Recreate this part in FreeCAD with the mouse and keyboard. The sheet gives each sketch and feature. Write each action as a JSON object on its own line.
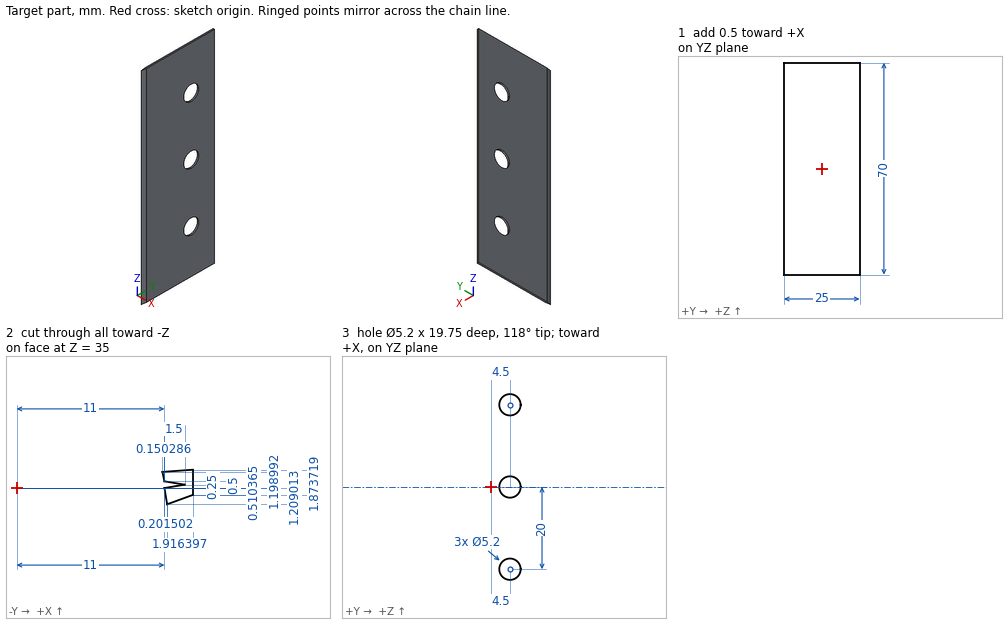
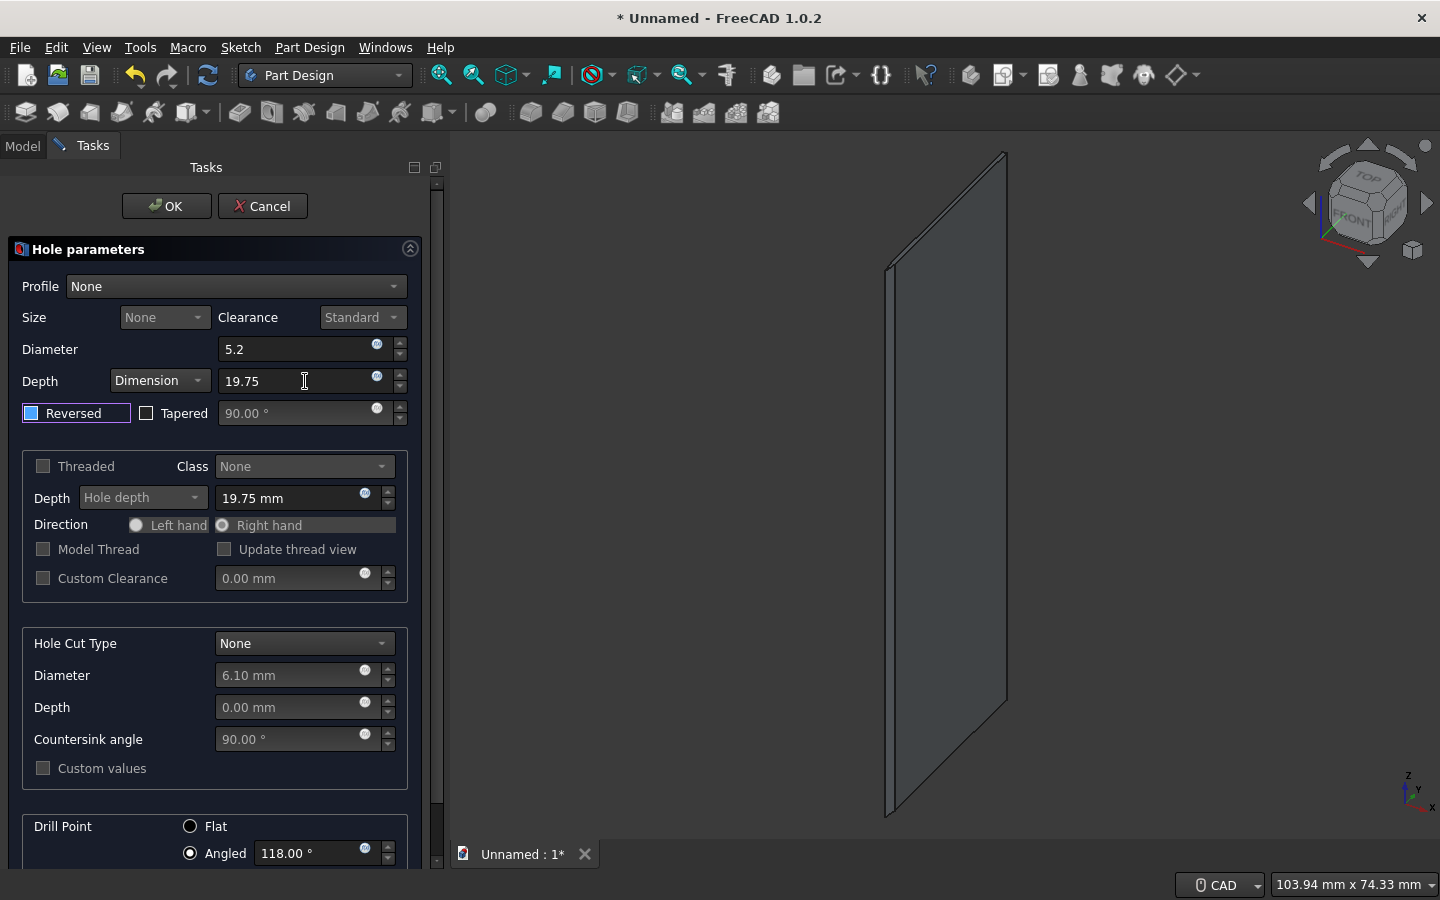
{"action": "left_click", "coordinate": [30, 413]}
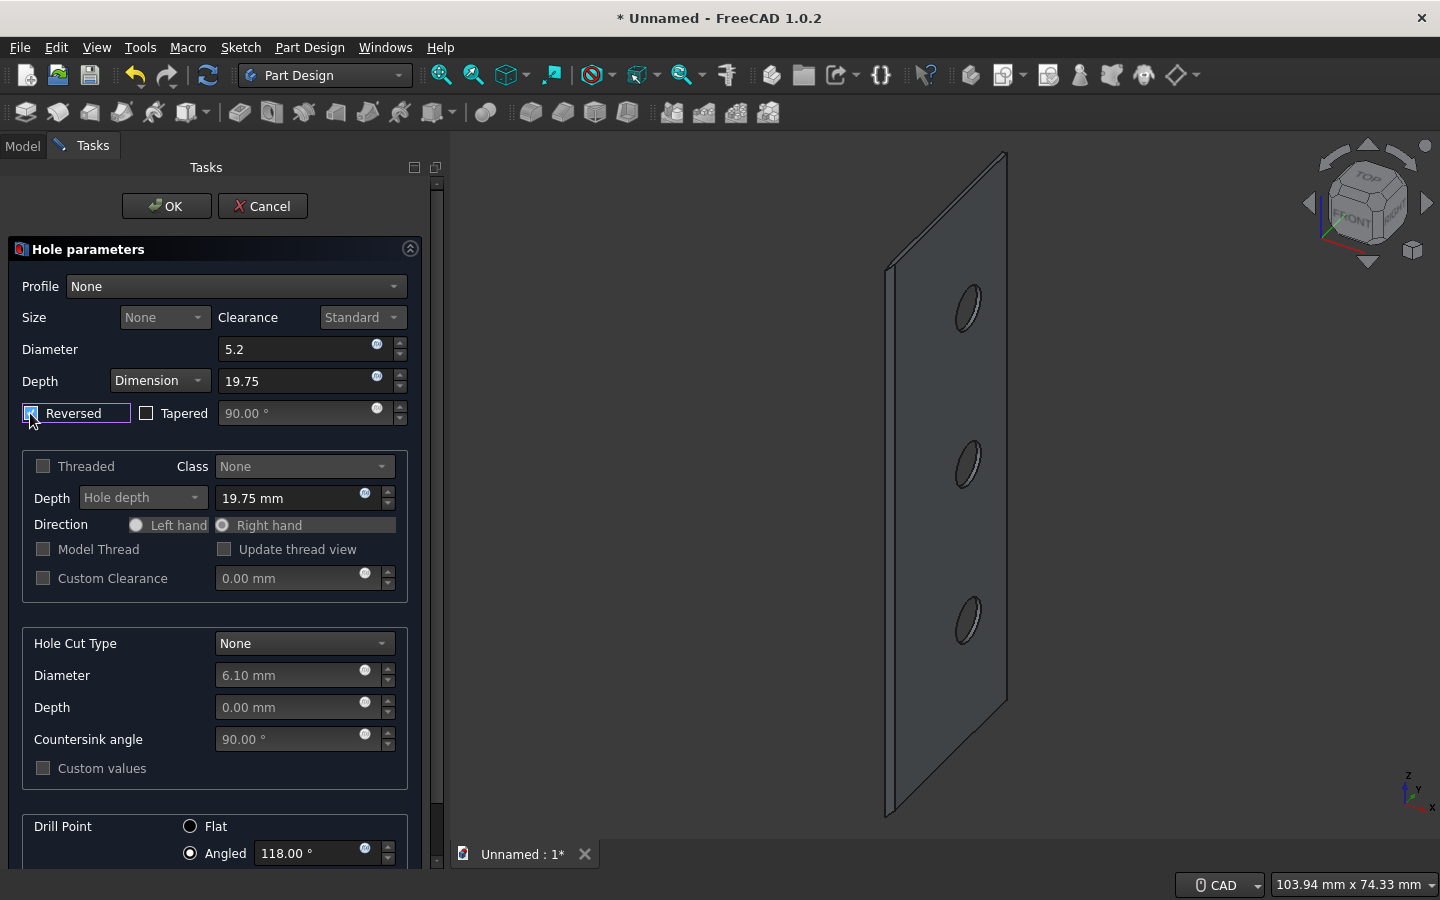
{"action": "left_click", "coordinate": [167, 206]}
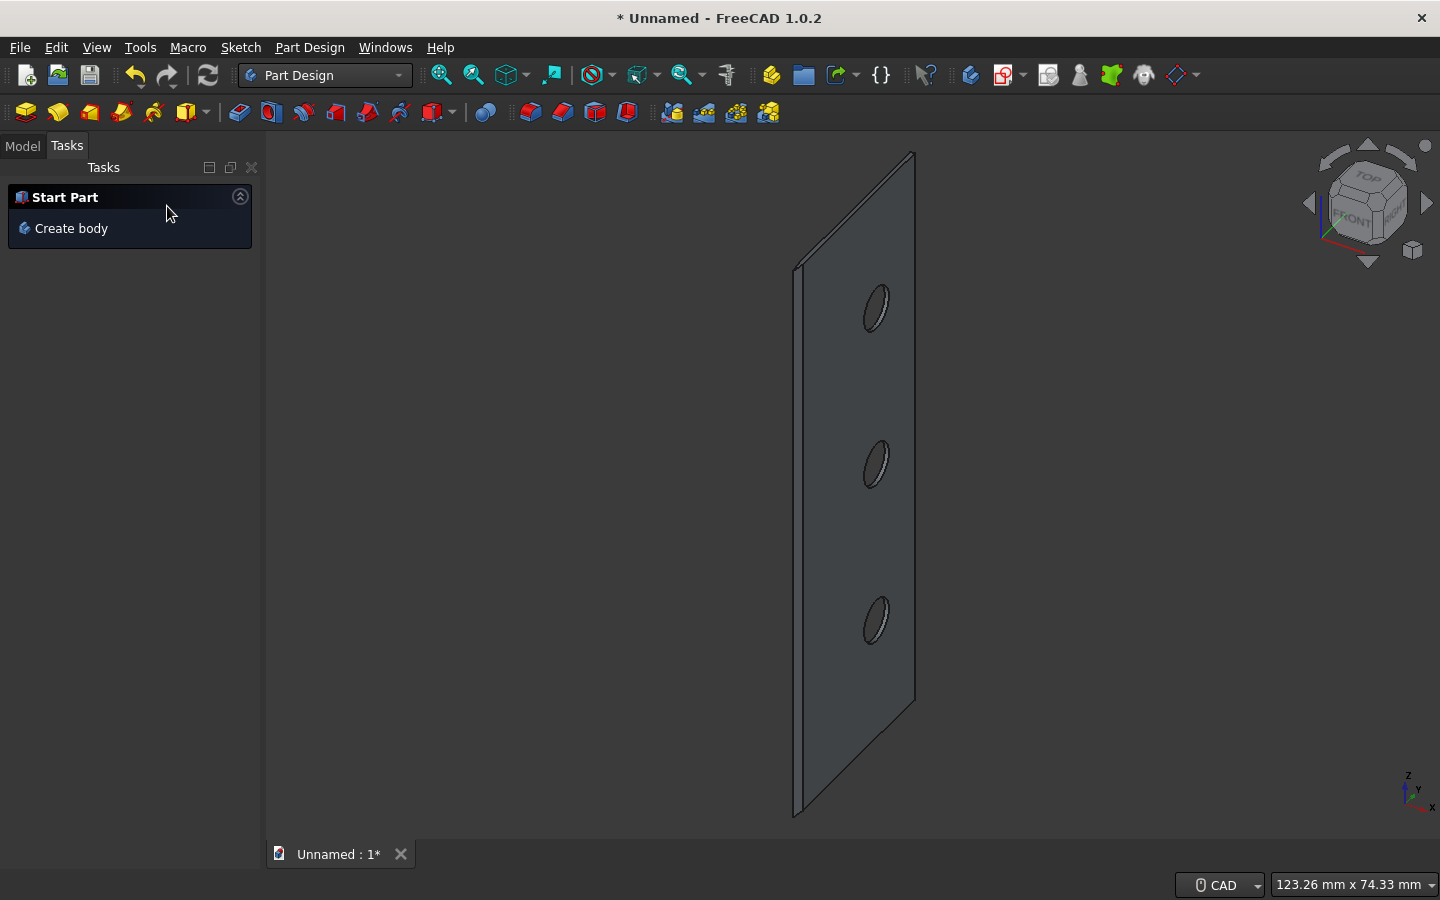
{"action": "key", "text": "0"}